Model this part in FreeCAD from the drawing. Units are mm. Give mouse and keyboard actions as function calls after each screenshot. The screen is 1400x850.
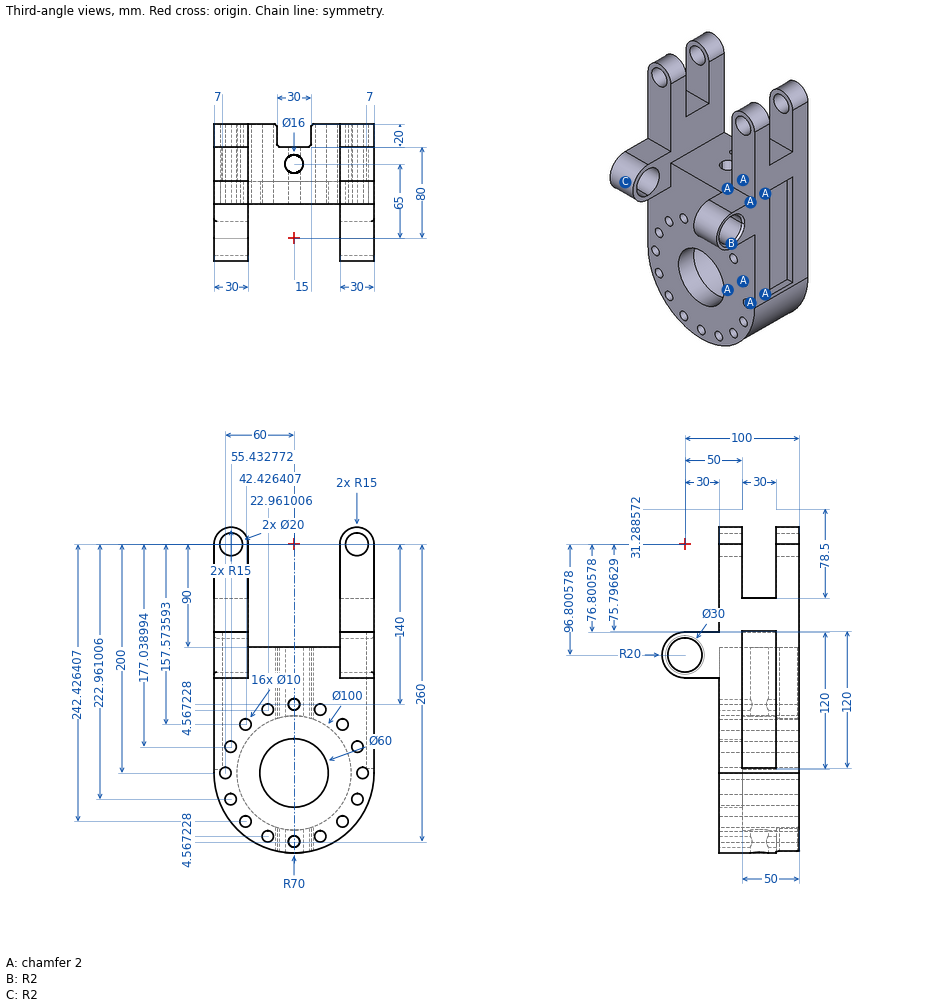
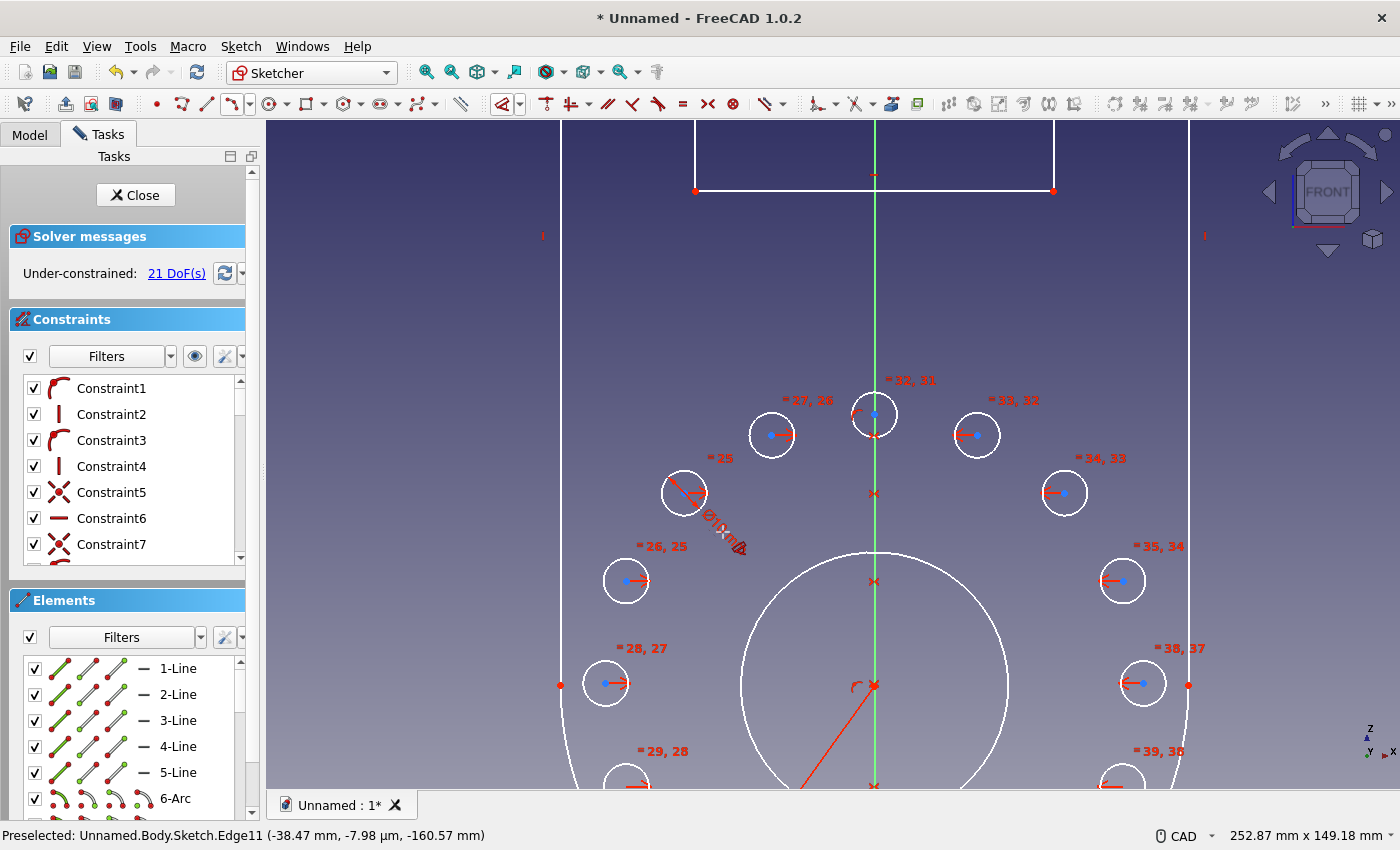
click(969, 591)
click(992, 568)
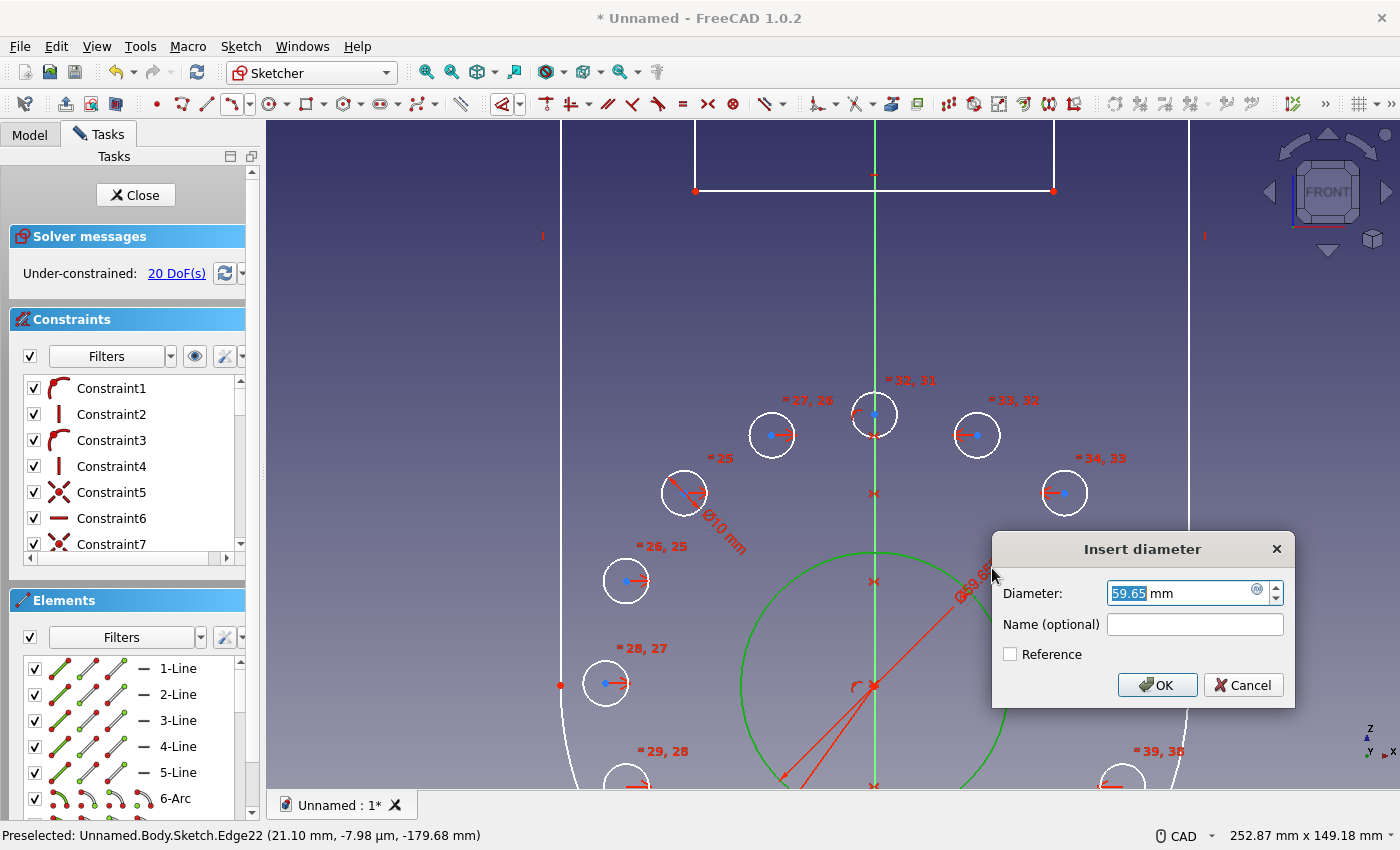
text(60)
key(Return)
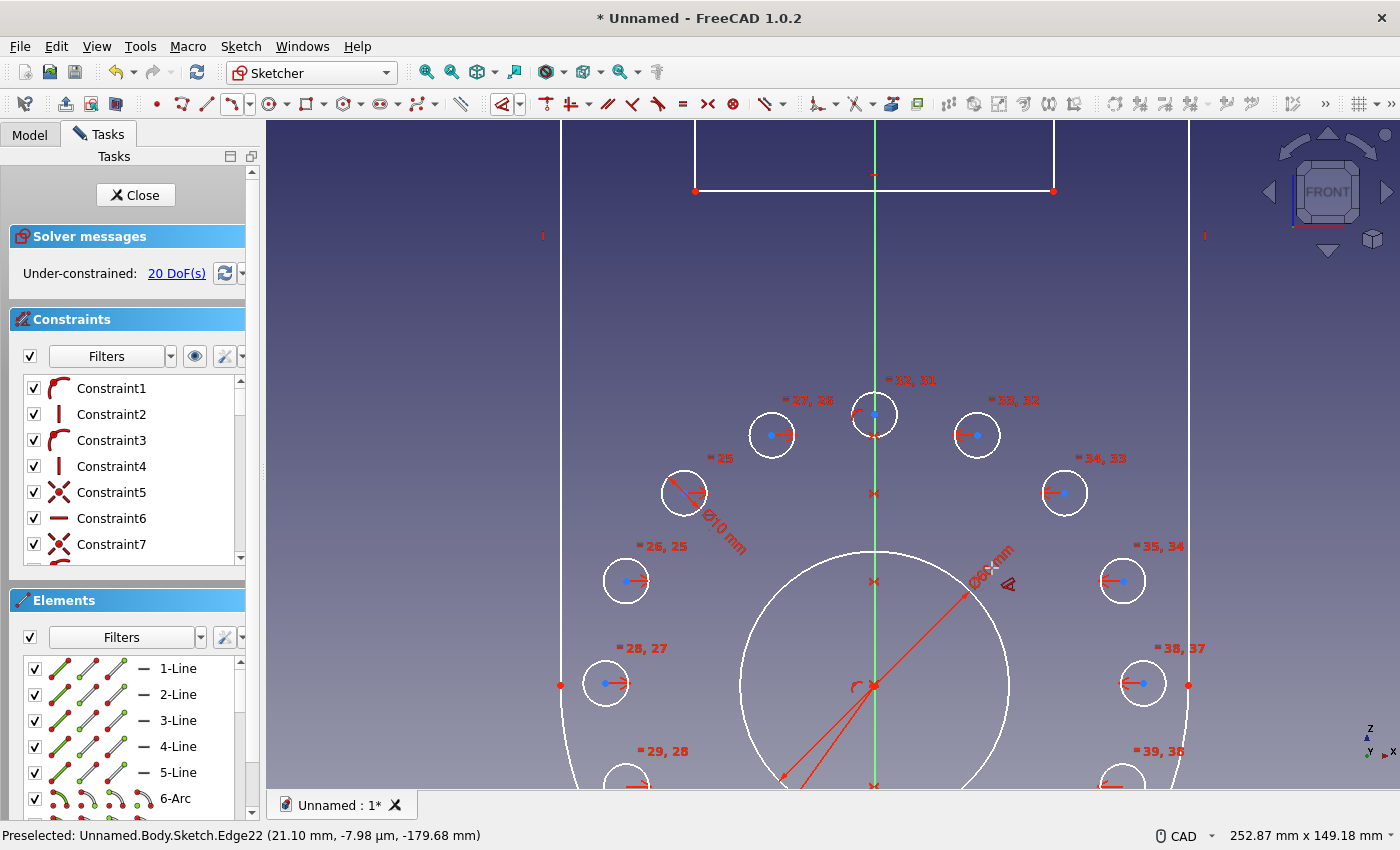
scroll(700, 511, down, 5)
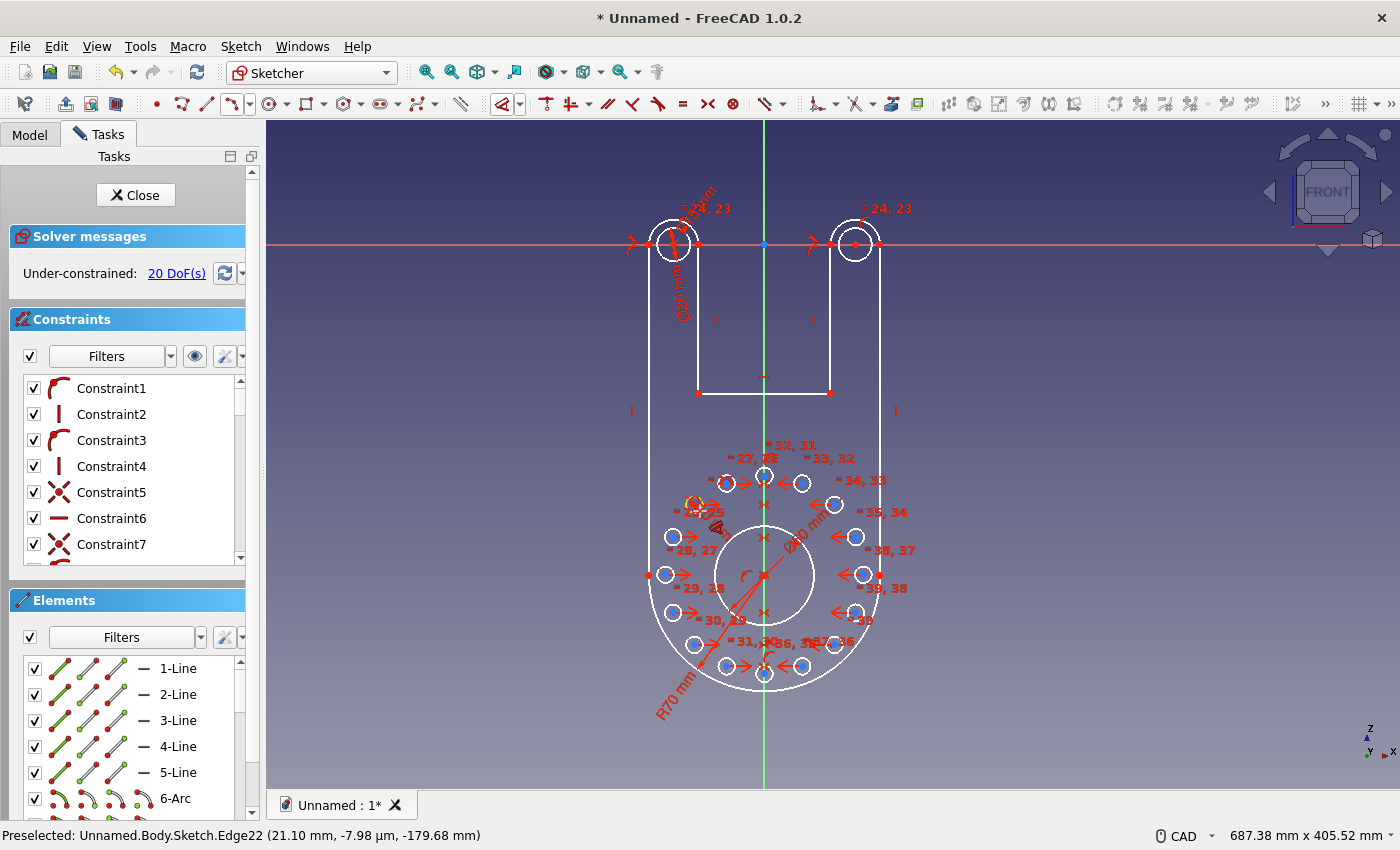
click(698, 289)
click(664, 319)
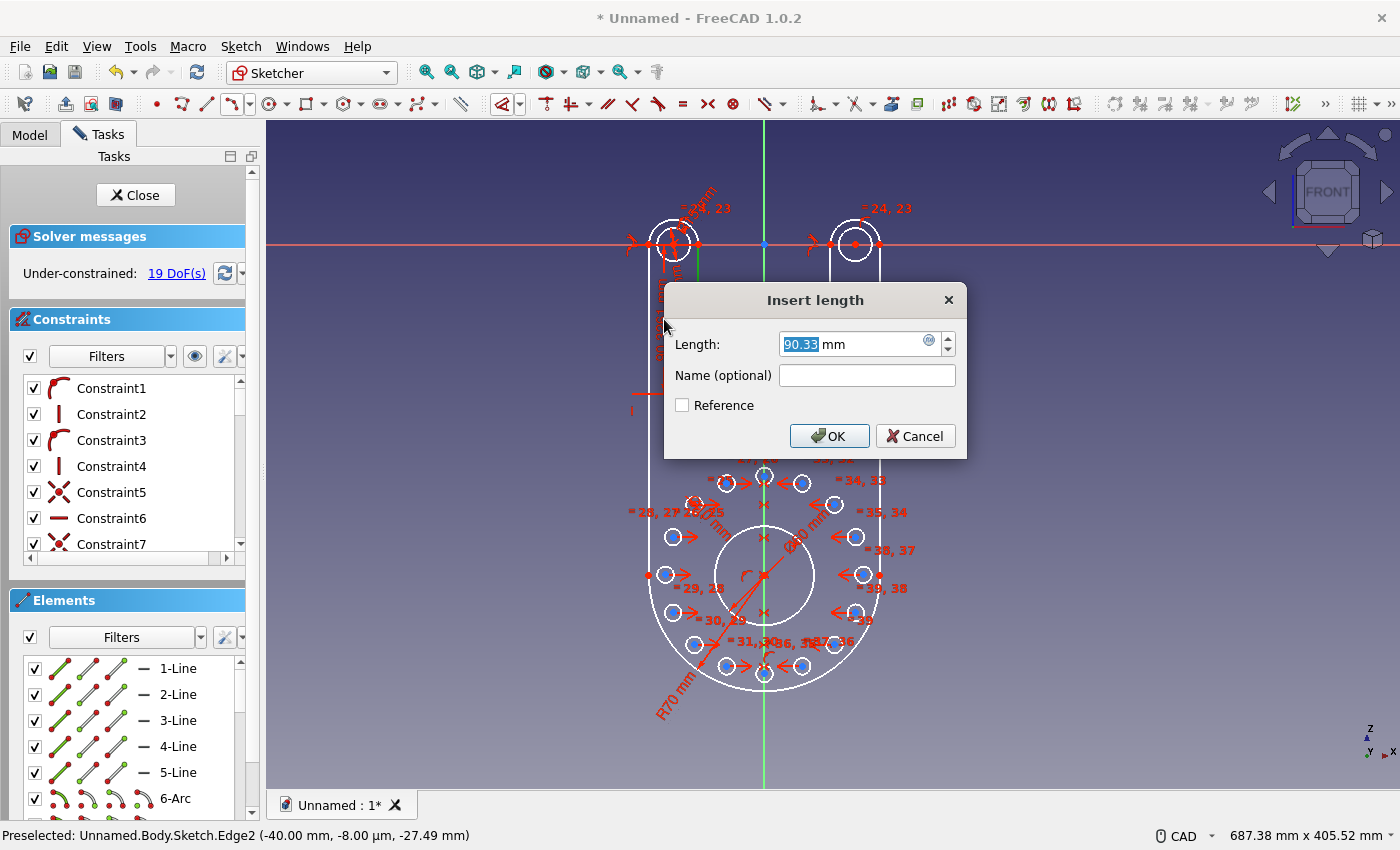
text(90)
key(Return)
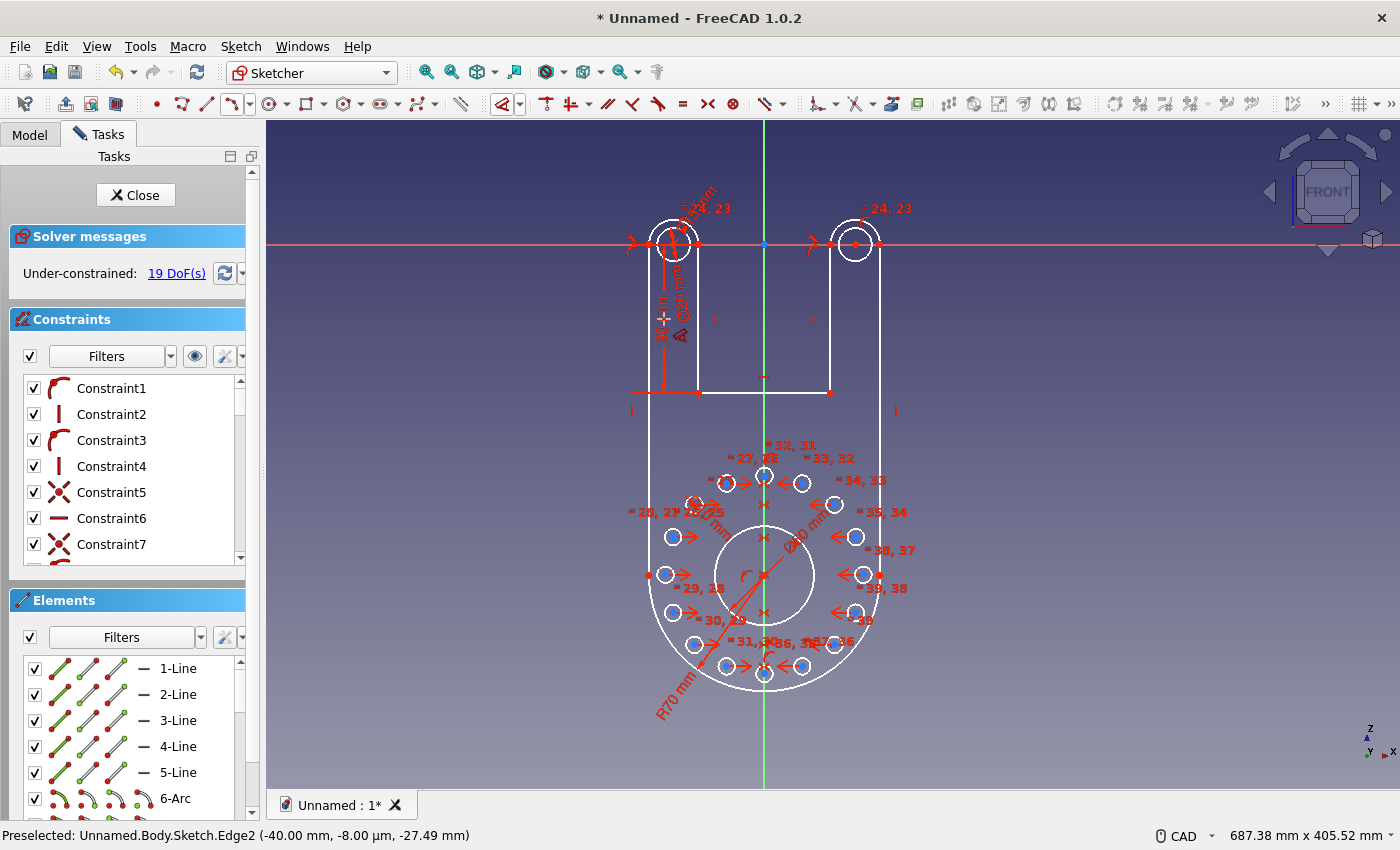
click(666, 575)
click(750, 609)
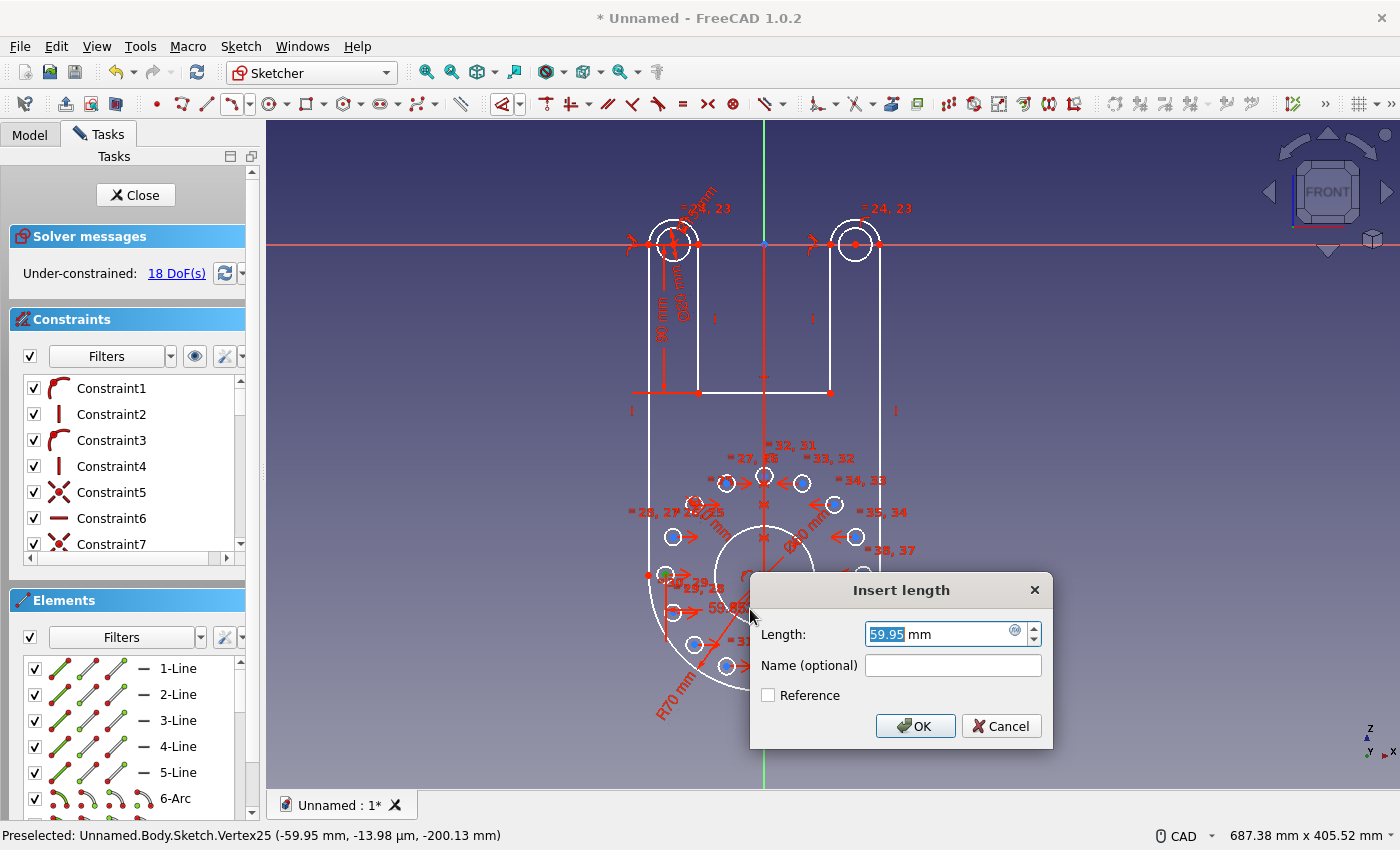
text(60)
key(Return)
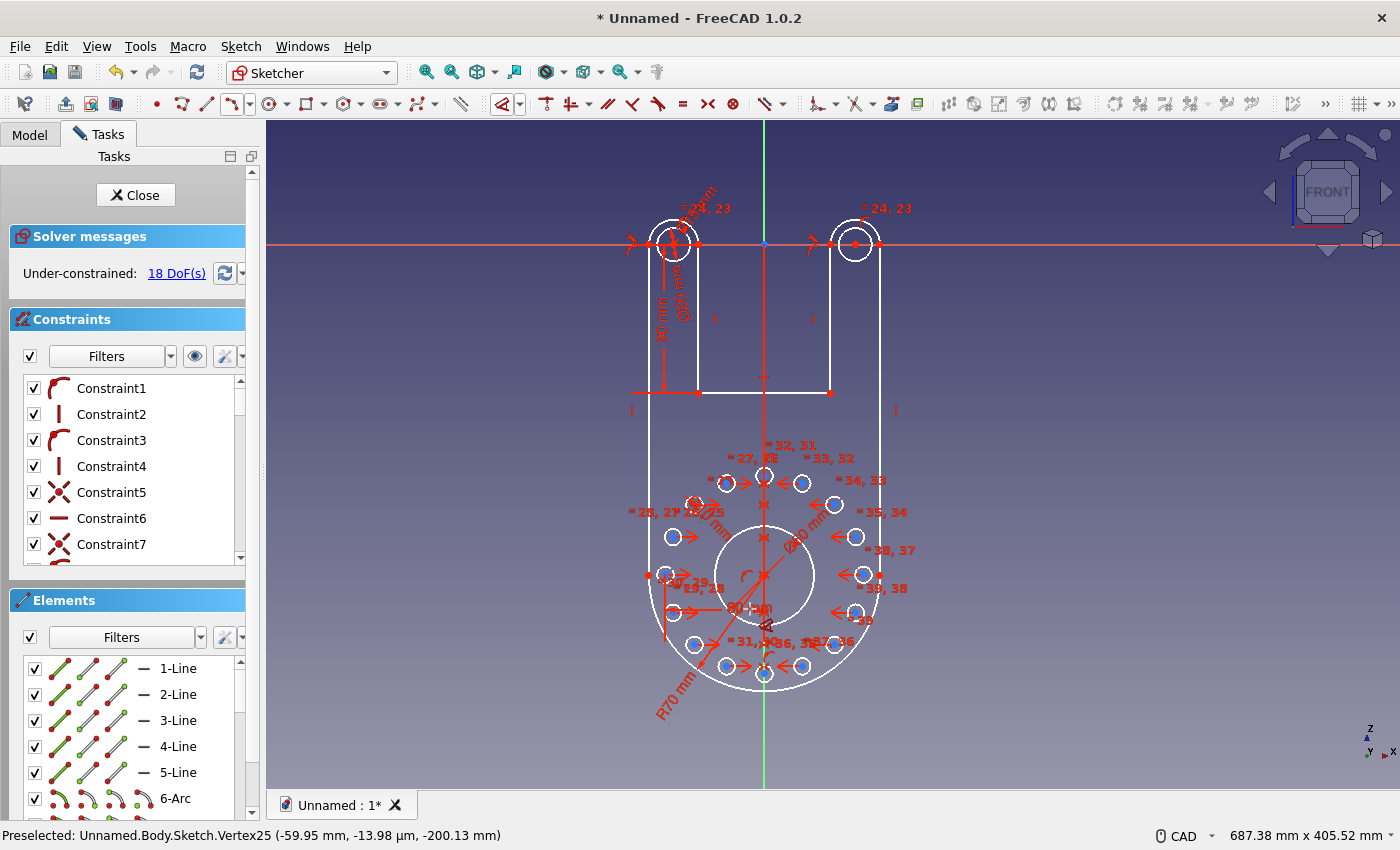
click(649, 476)
click(615, 410)